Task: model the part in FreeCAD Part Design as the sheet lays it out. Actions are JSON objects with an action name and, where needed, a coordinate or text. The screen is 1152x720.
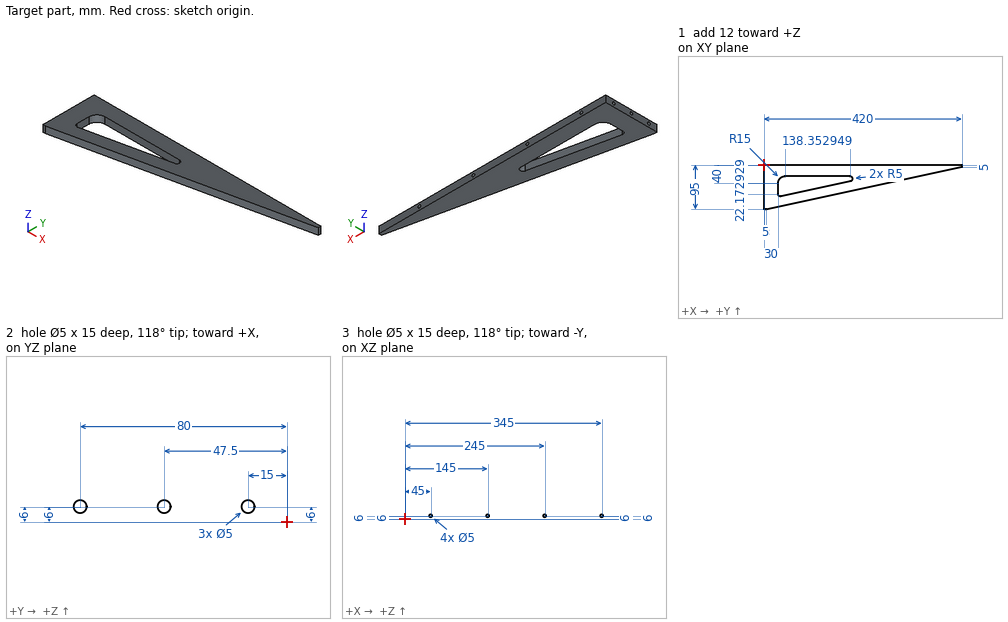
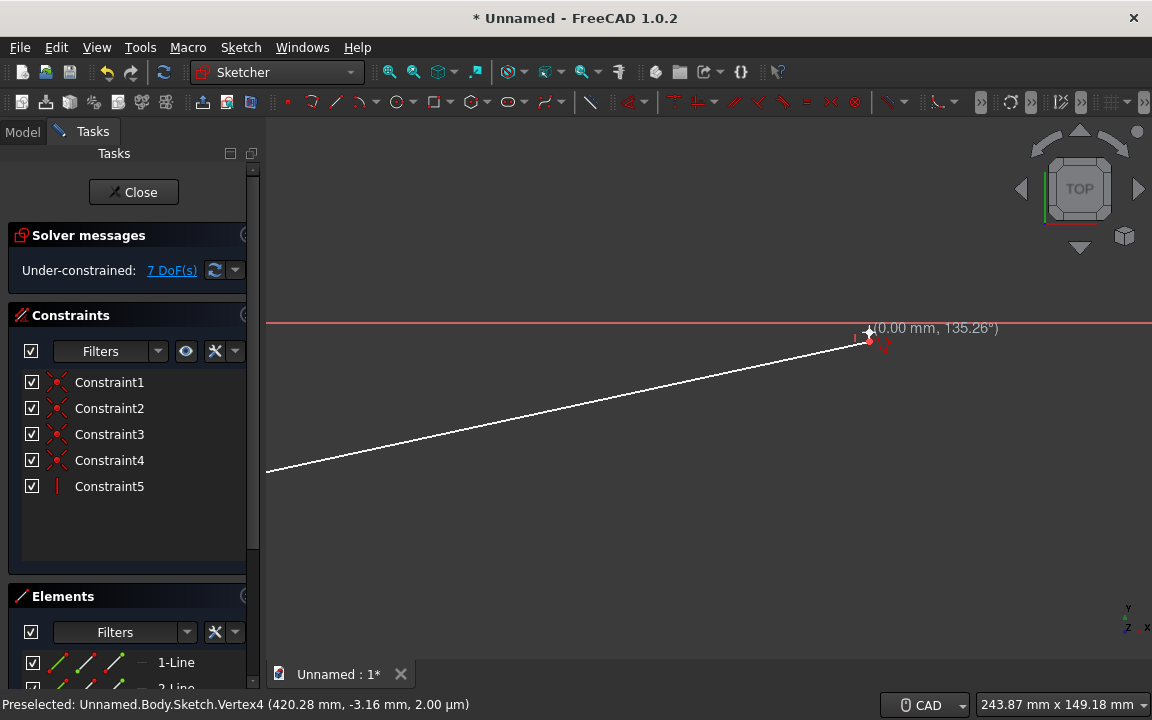
{"action": "scroll", "coordinate": [871, 342], "scroll_direction": "down", "scroll_amount": 6}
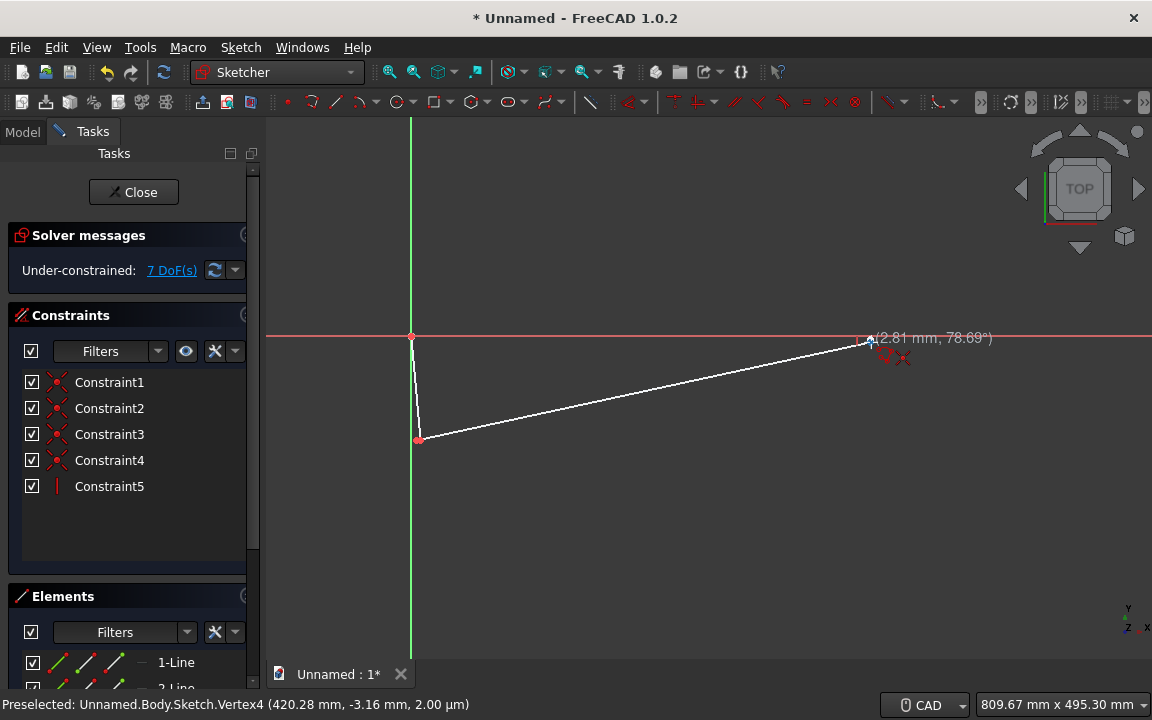
{"action": "left_click", "coordinate": [411, 336]}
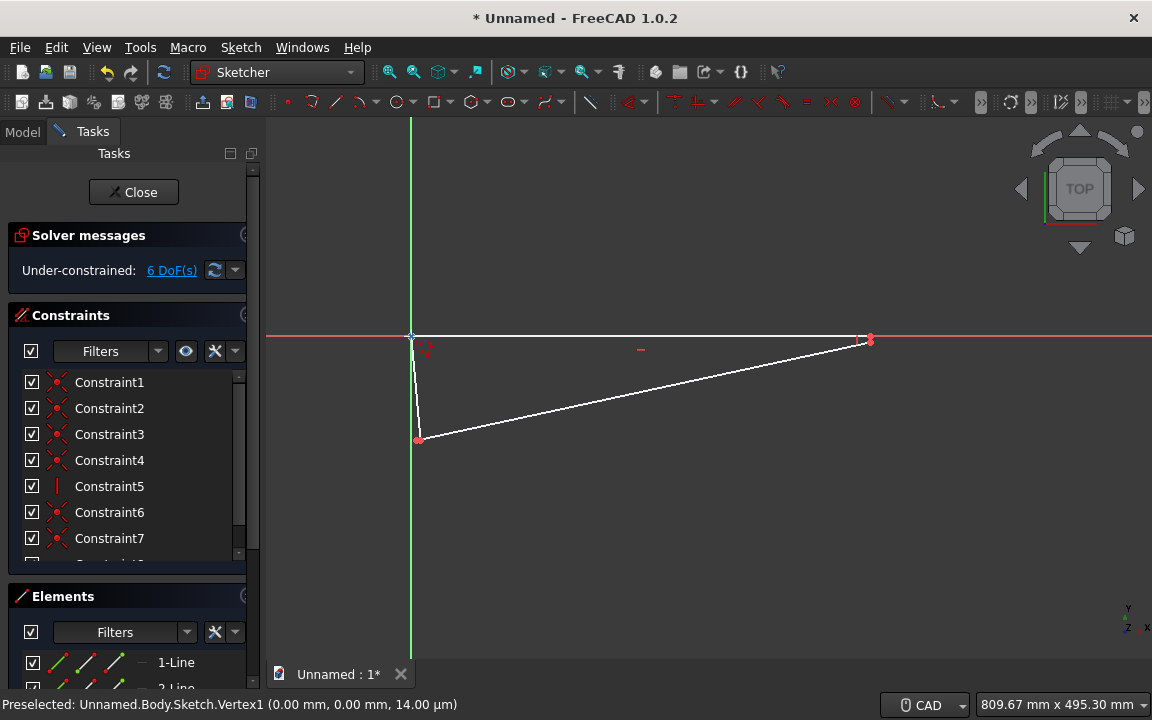
{"action": "left_click", "coordinate": [336, 102]}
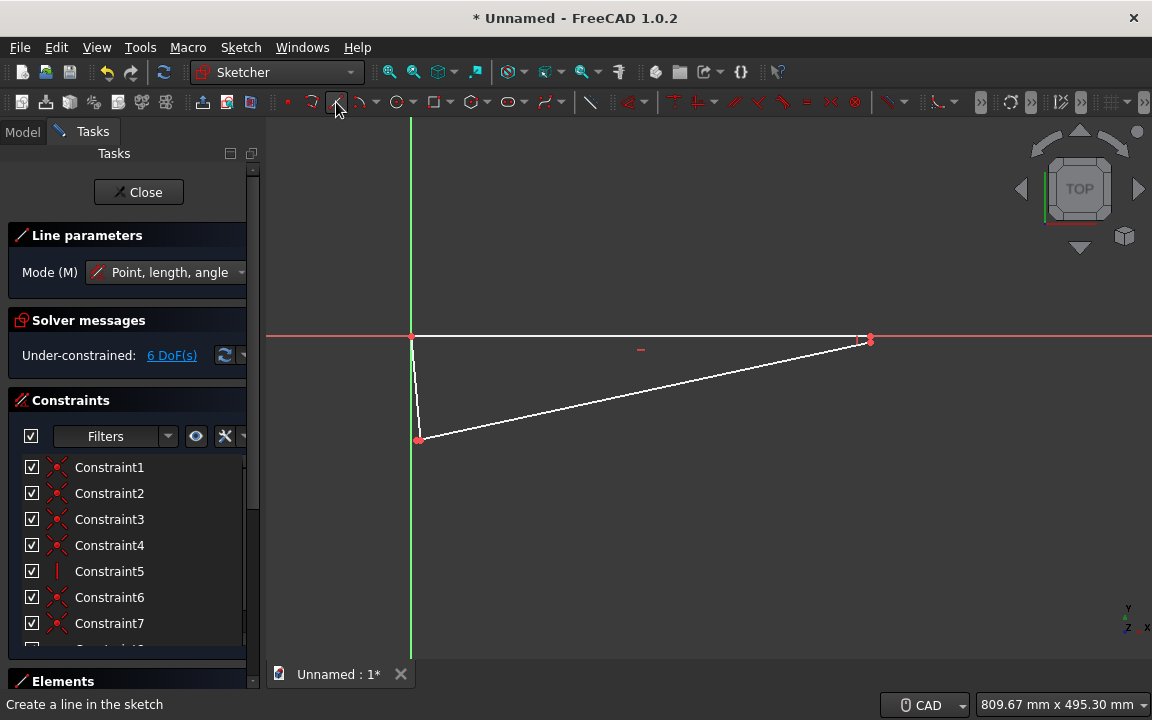
{"action": "left_click", "coordinate": [444, 404]}
{"action": "left_click", "coordinate": [444, 380]}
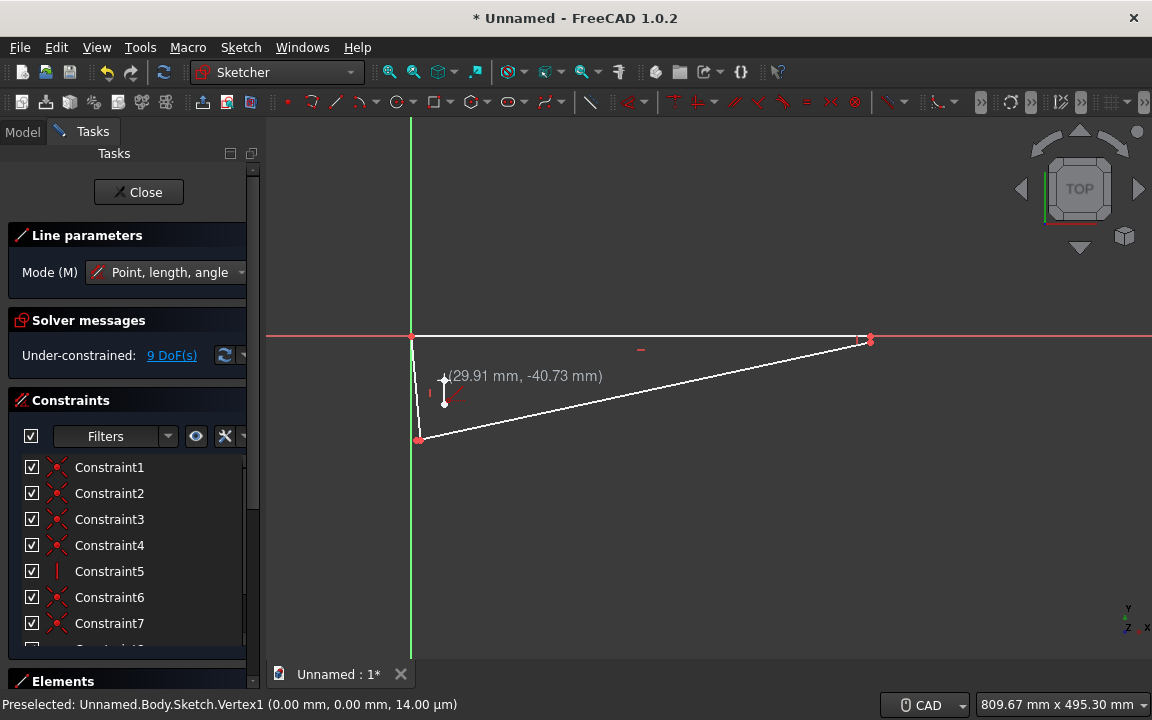
{"action": "left_click", "coordinate": [461, 364]}
{"action": "left_click", "coordinate": [612, 364]}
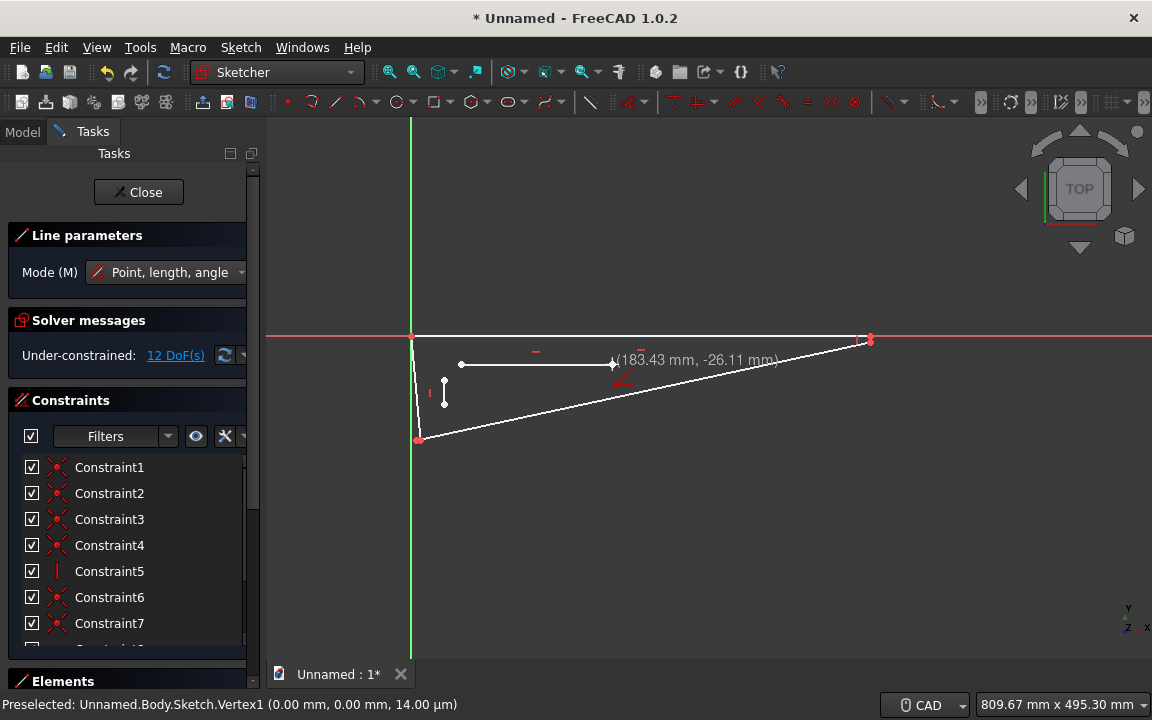
{"action": "scroll", "coordinate": [613, 375], "scroll_direction": "up", "scroll_amount": 2}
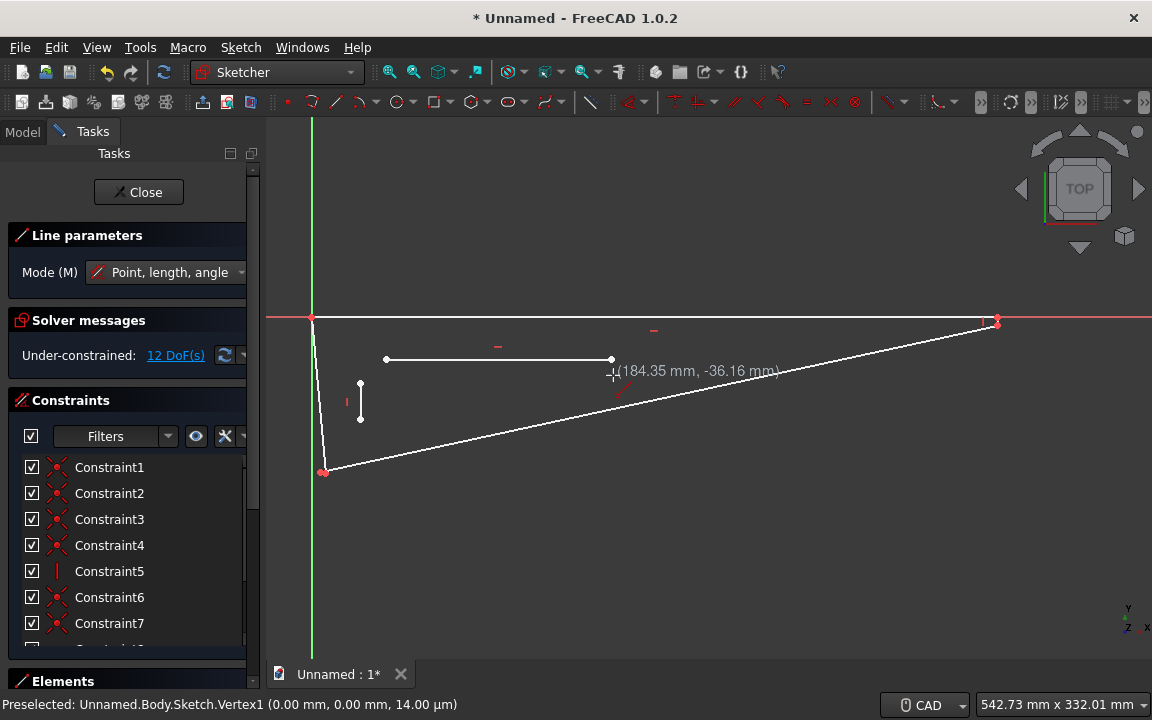
{"action": "left_click", "coordinate": [613, 374]}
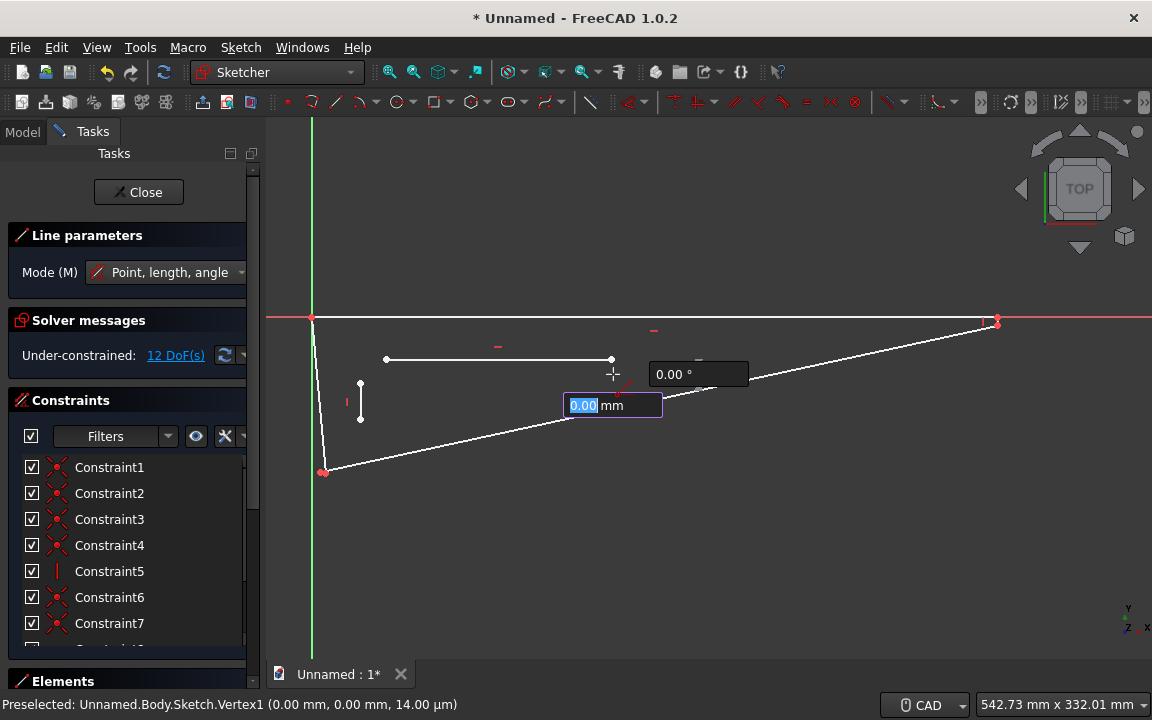
{"action": "scroll", "coordinate": [371, 427], "scroll_direction": "up", "scroll_amount": 2}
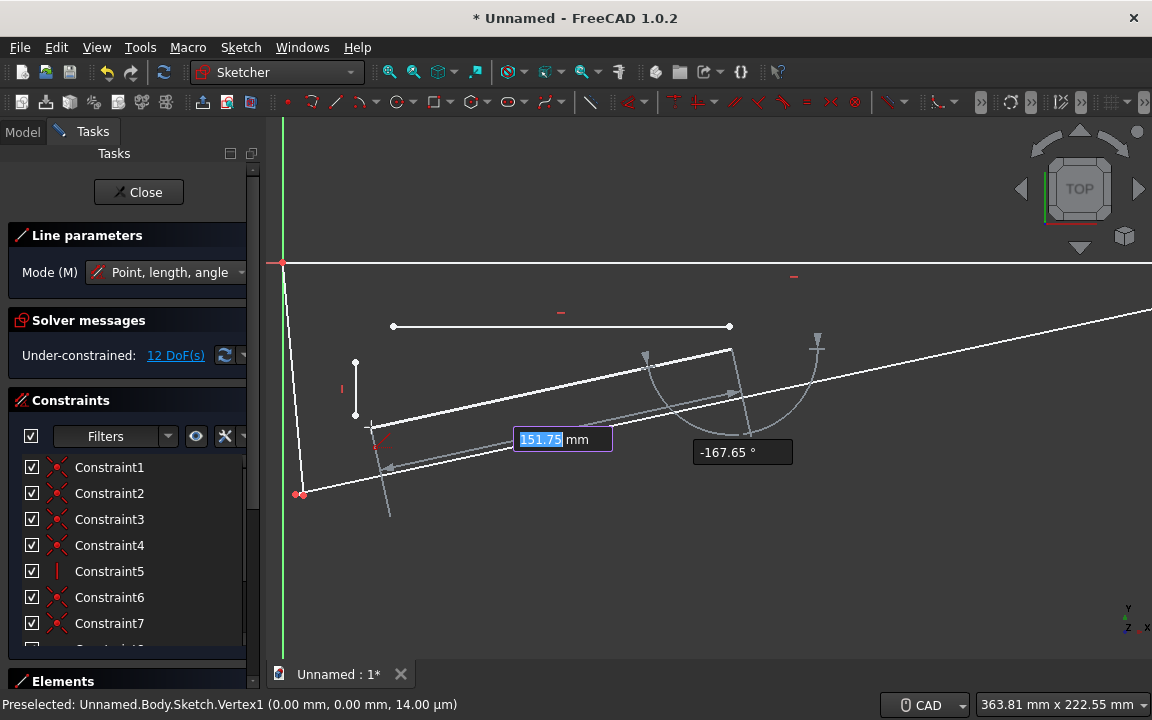
{"action": "left_click", "coordinate": [371, 426]}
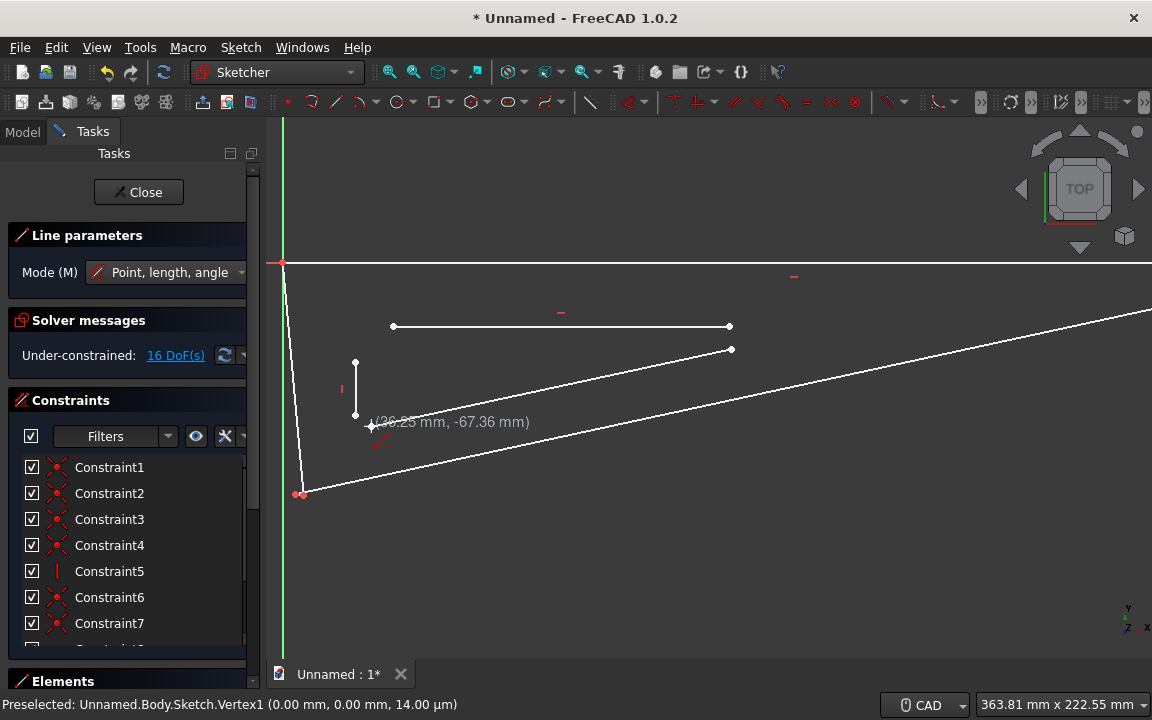
{"action": "left_click", "coordinate": [378, 102]}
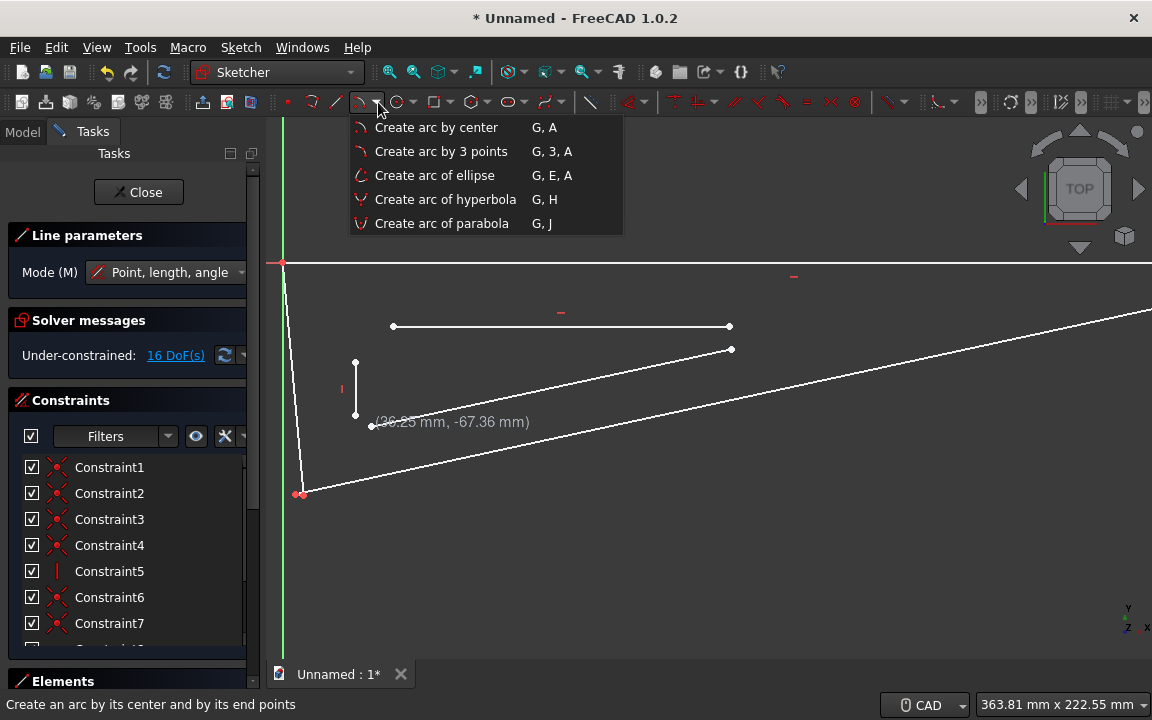
{"action": "left_click", "coordinate": [486, 151]}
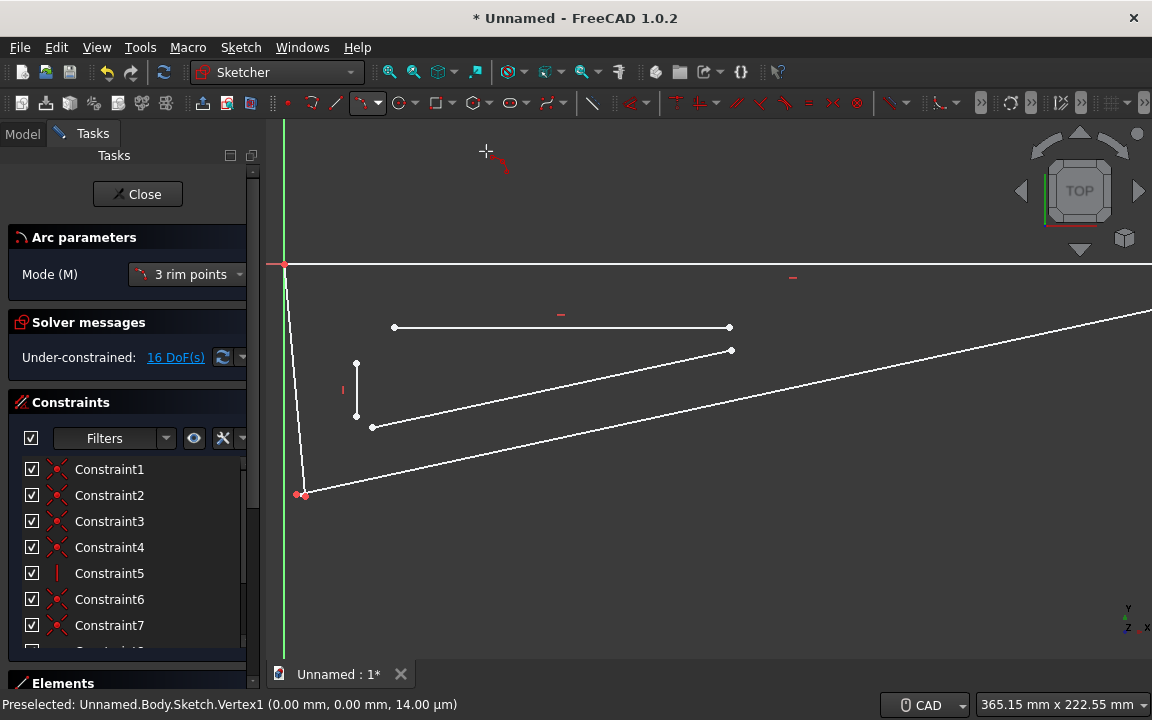
{"action": "left_click", "coordinate": [357, 363]}
{"action": "left_click", "coordinate": [395, 328]}